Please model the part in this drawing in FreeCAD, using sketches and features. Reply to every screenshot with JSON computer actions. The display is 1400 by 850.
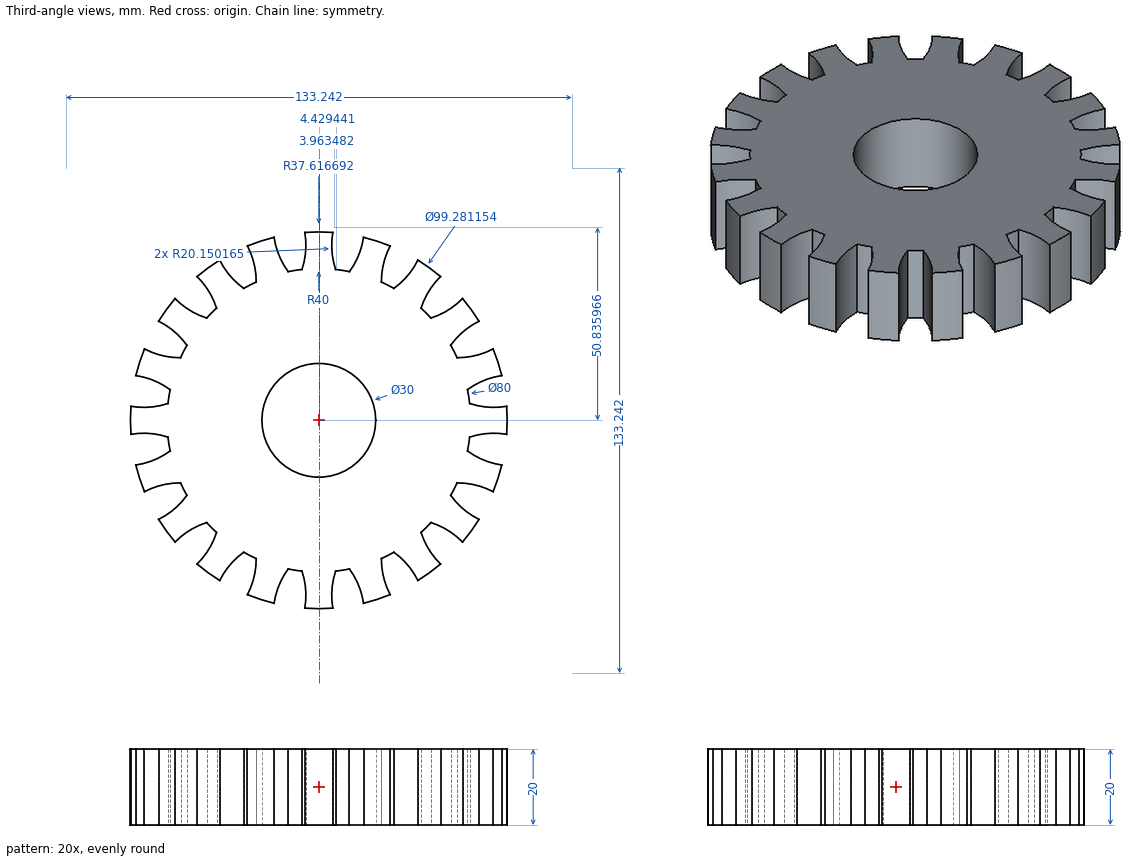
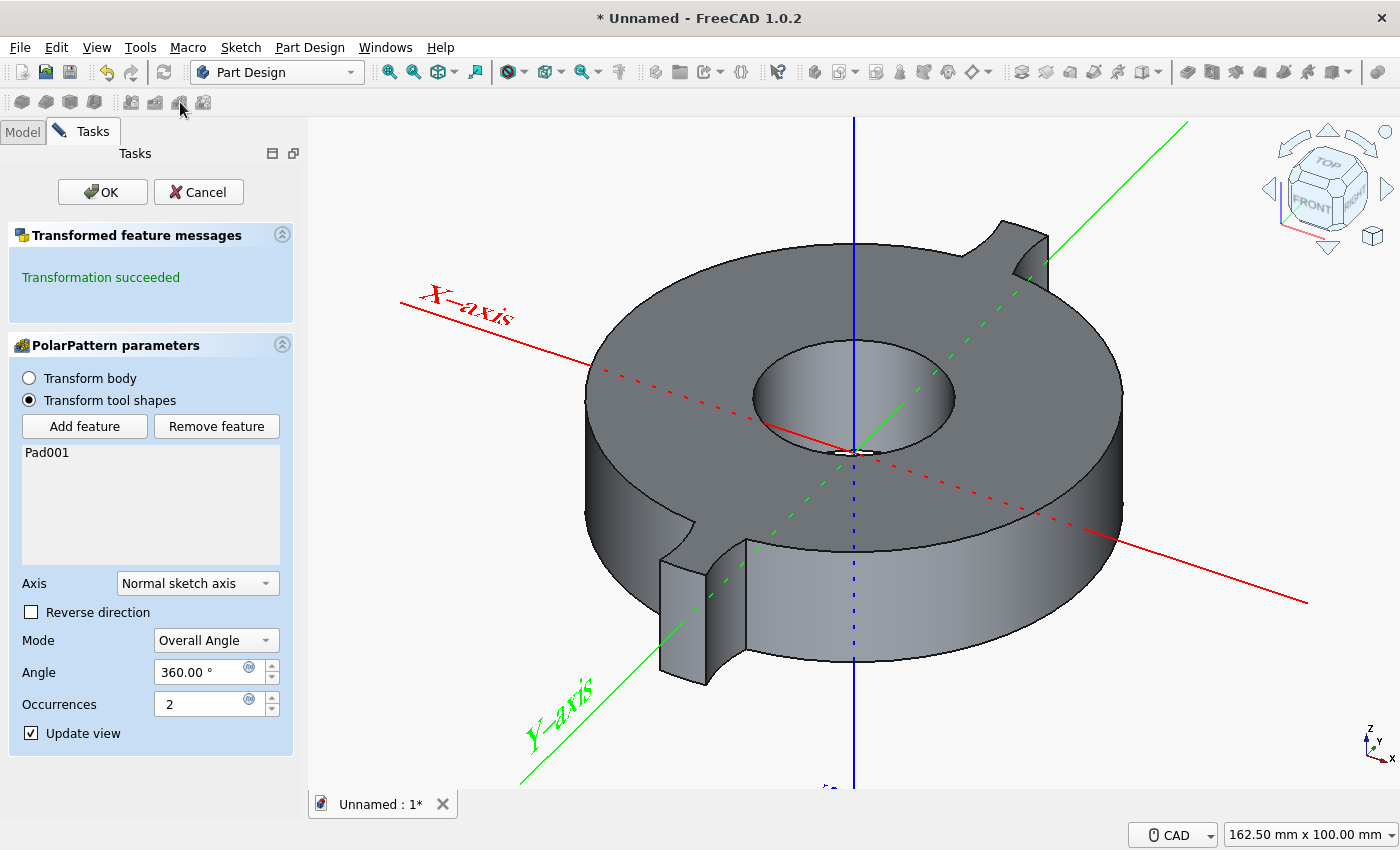
{"action": "left_click", "coordinate": [198, 584]}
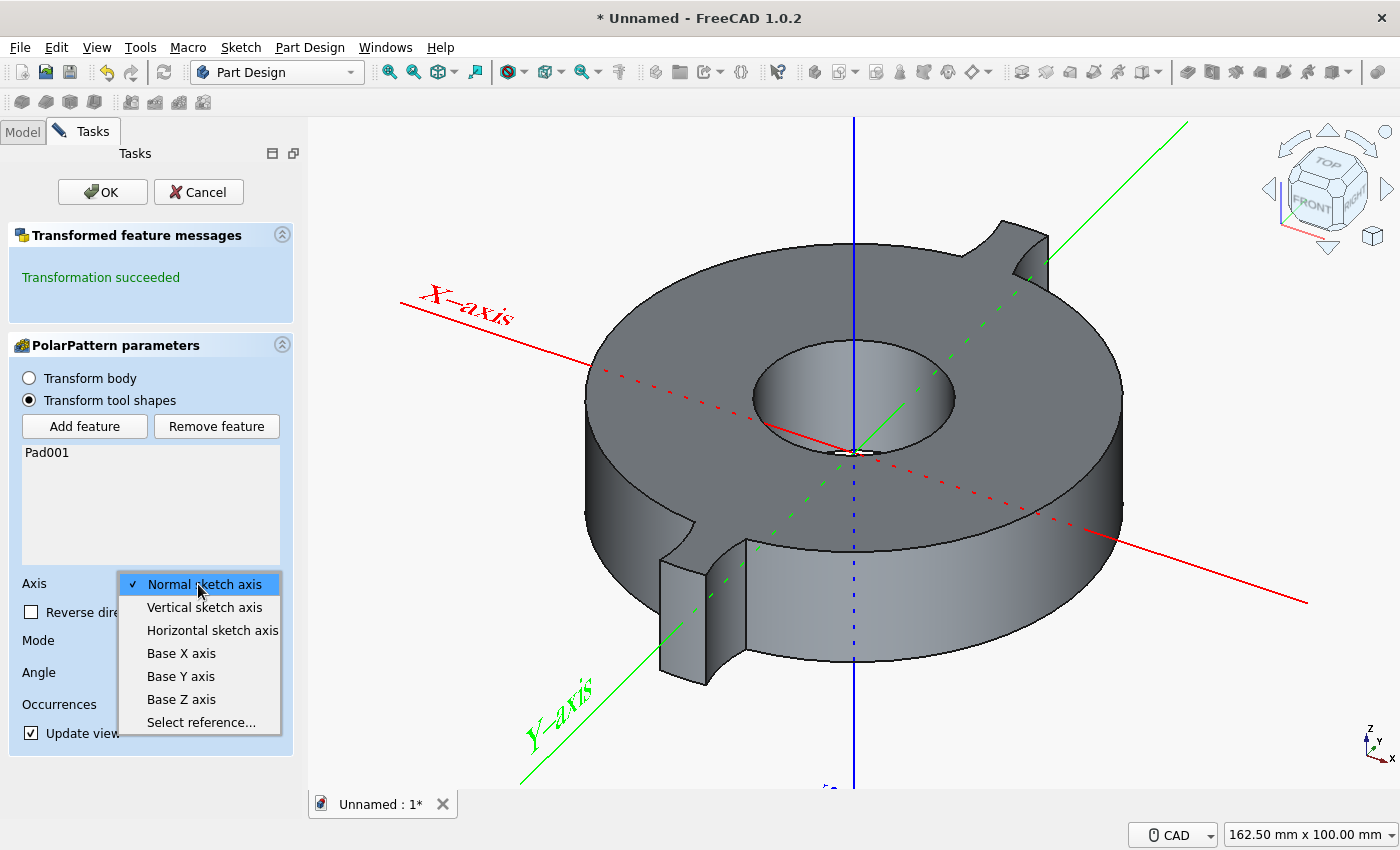
{"action": "left_click", "coordinate": [198, 700]}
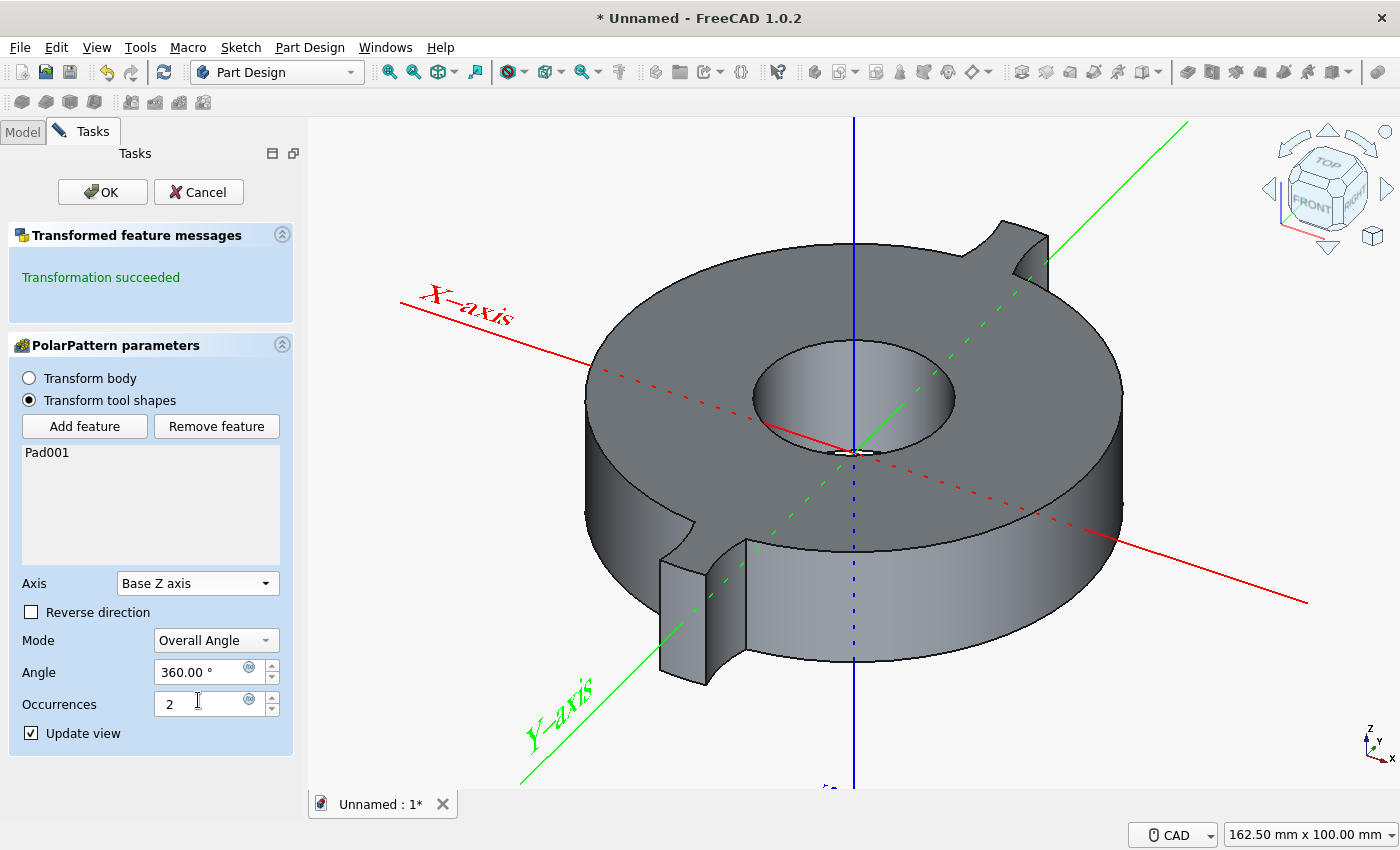
{"action": "triple_click", "coordinate": [209, 704]}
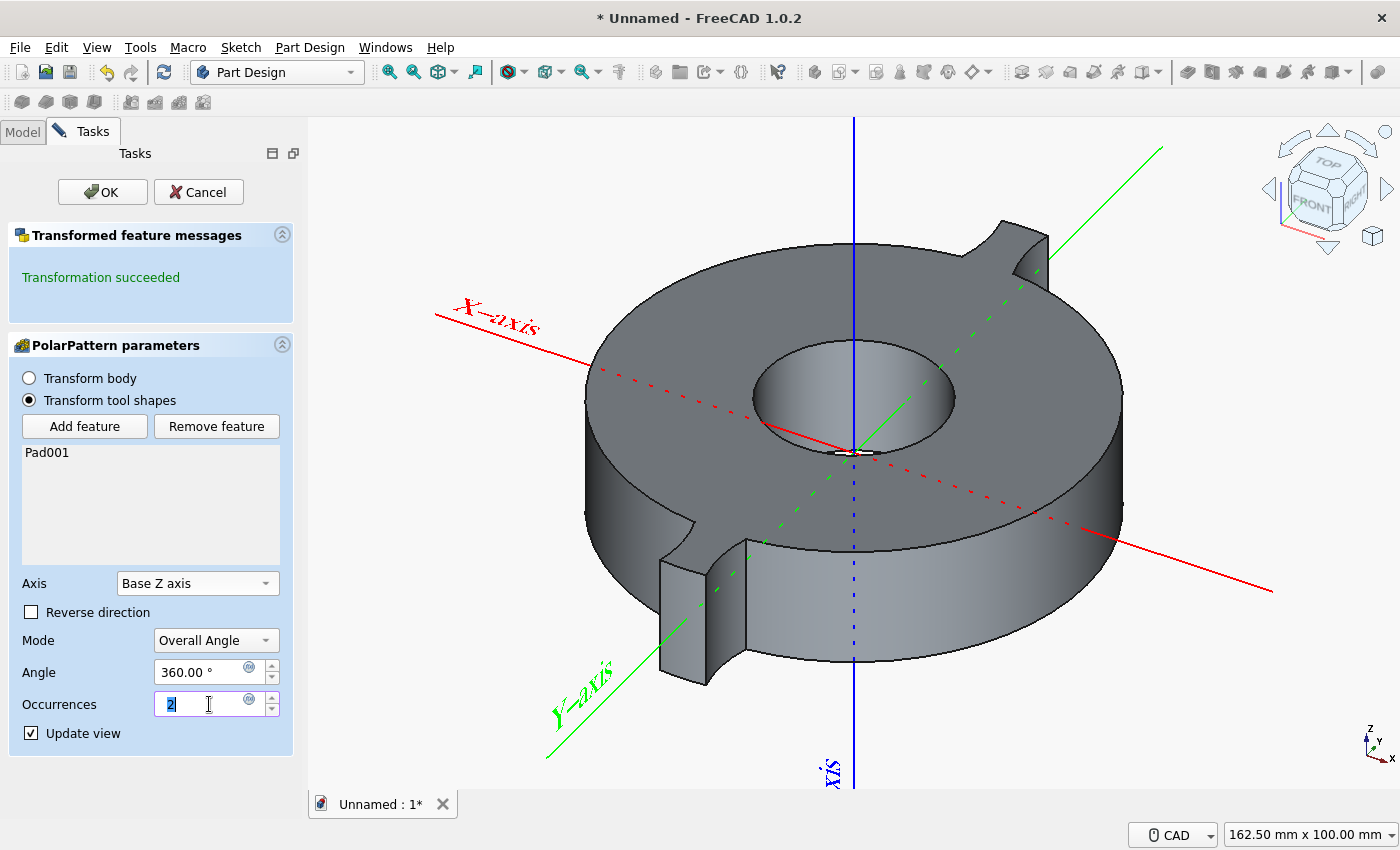
{"action": "type", "text": "20"}
{"action": "key", "text": "Tab"}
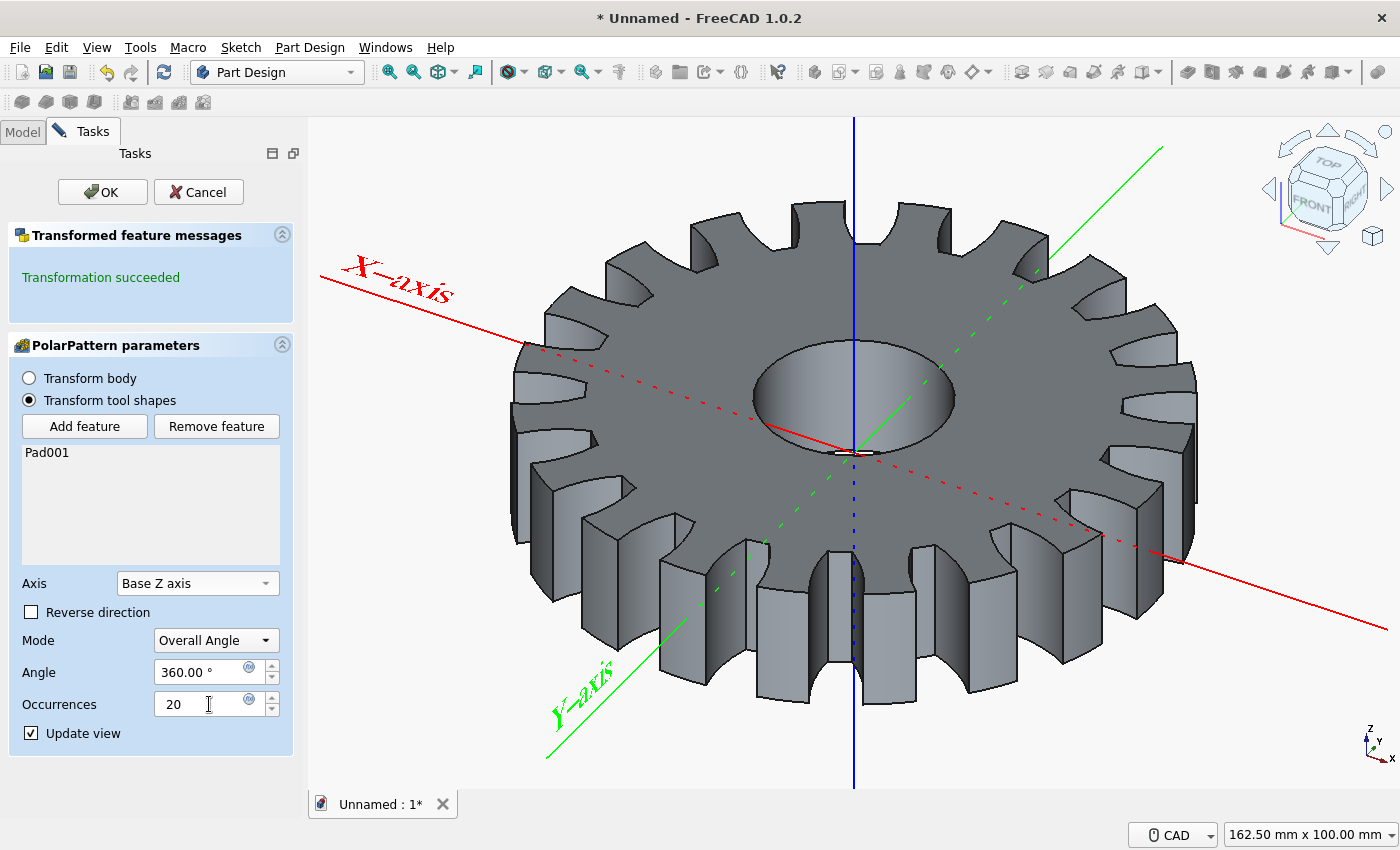
{"action": "left_click", "coordinate": [103, 192]}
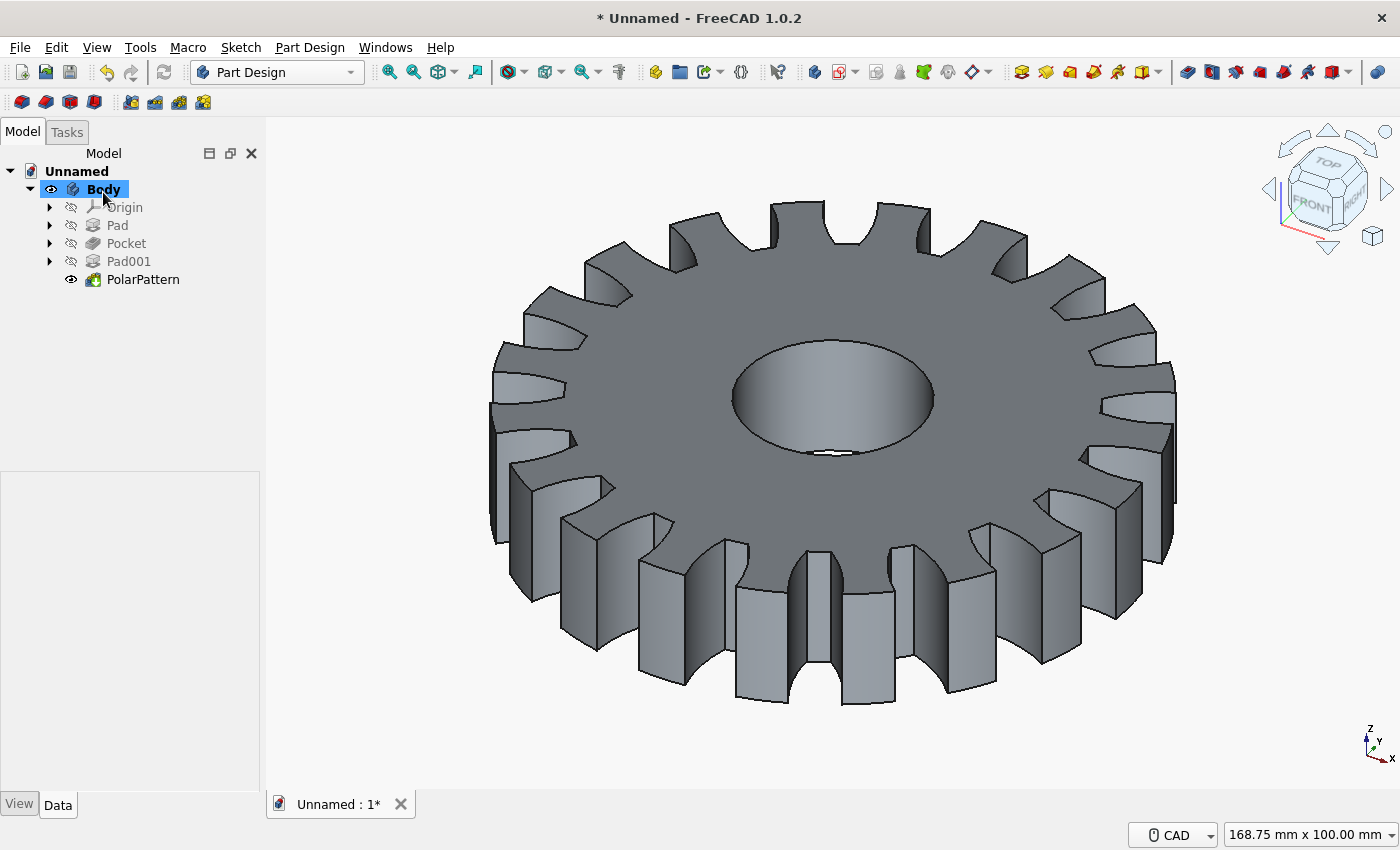
{"action": "key", "text": "5"}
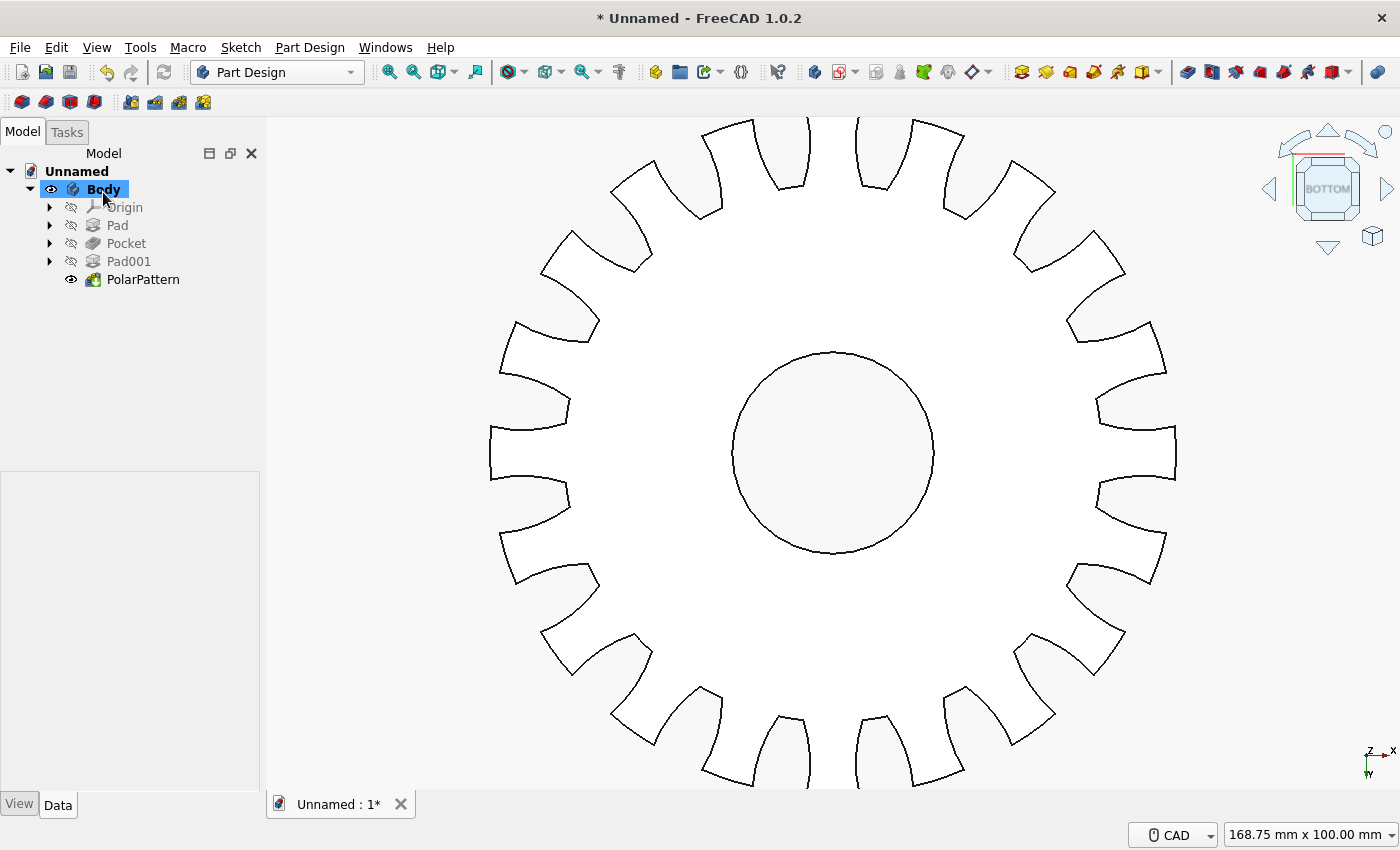
{"action": "key", "text": "v f"}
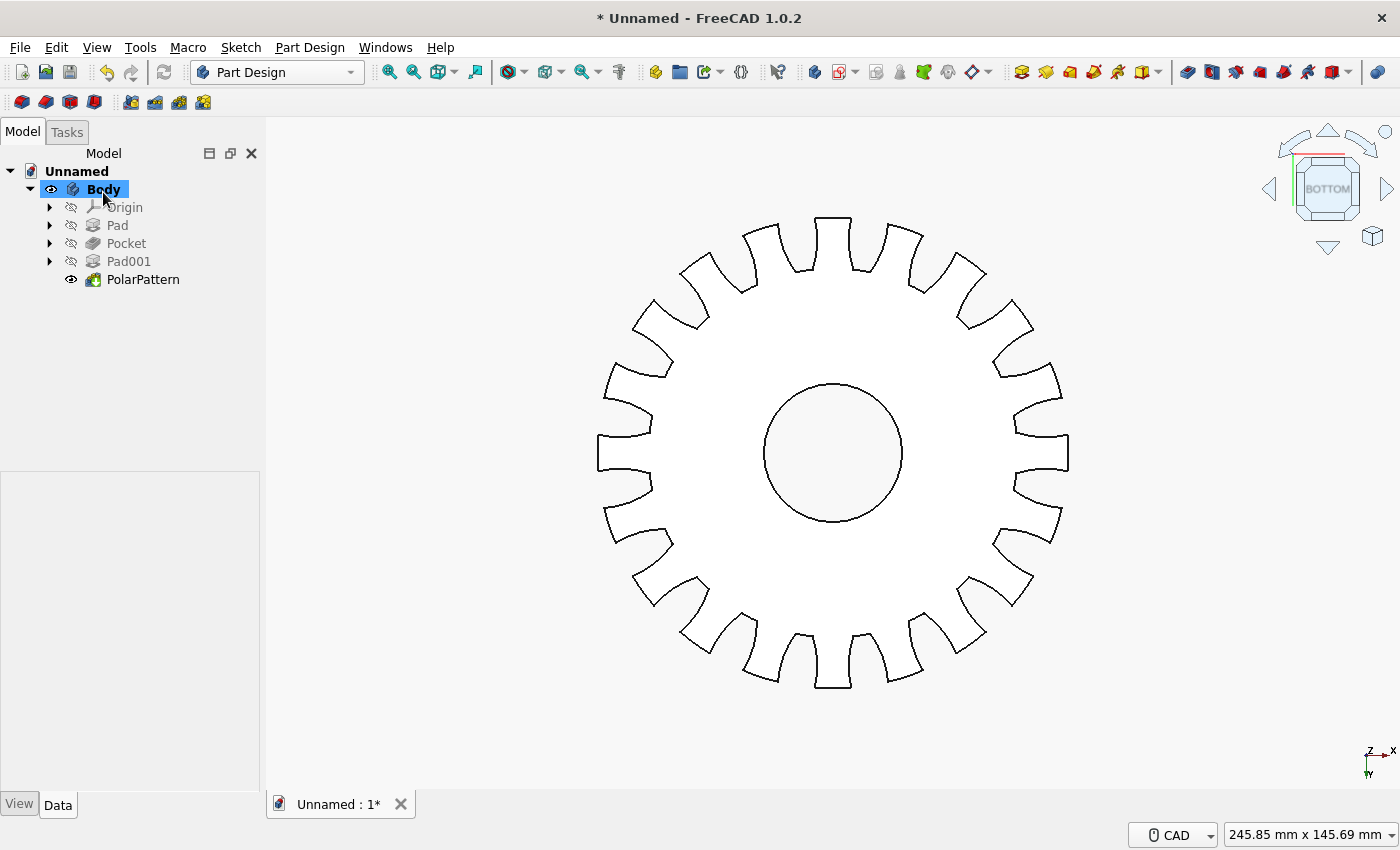
{"action": "left_click", "coordinate": [833, 587]}